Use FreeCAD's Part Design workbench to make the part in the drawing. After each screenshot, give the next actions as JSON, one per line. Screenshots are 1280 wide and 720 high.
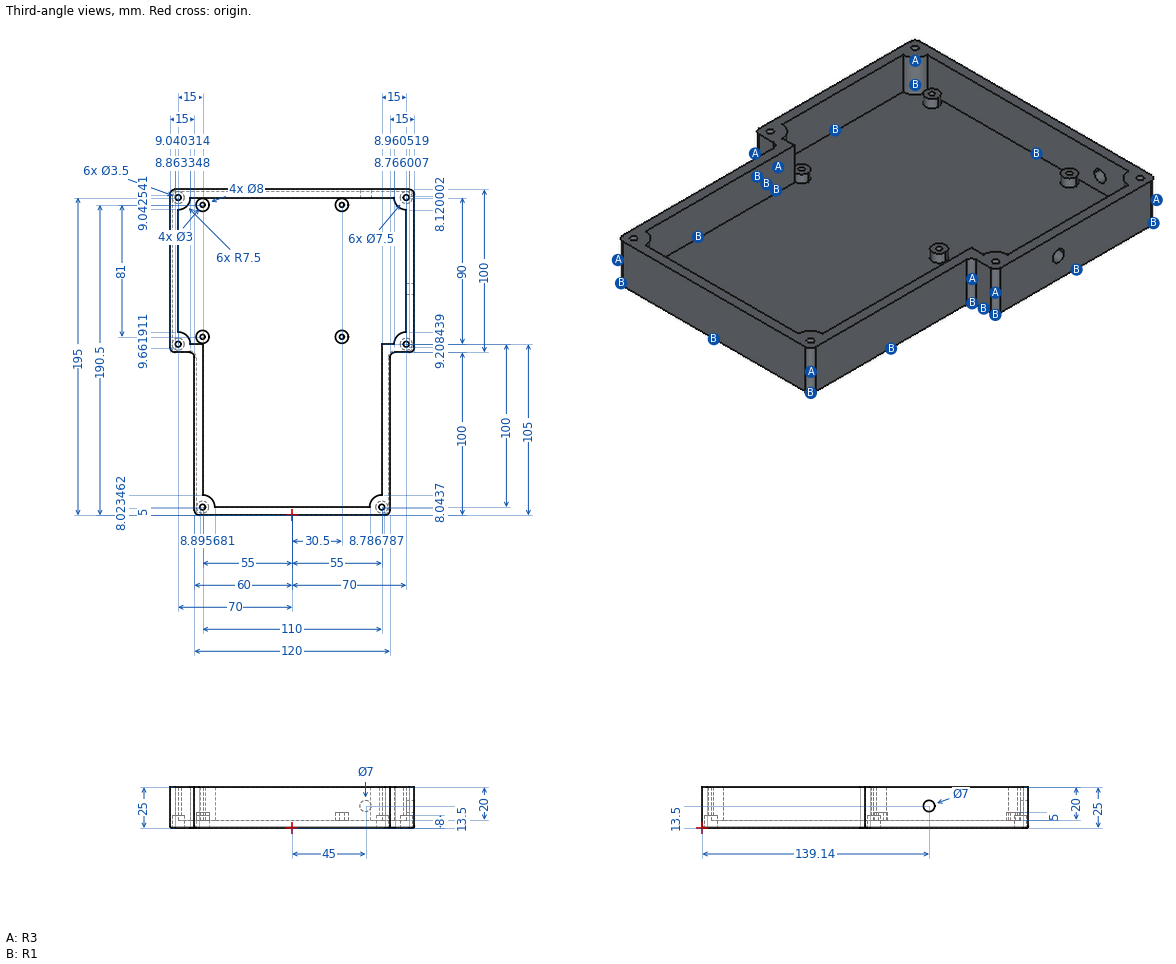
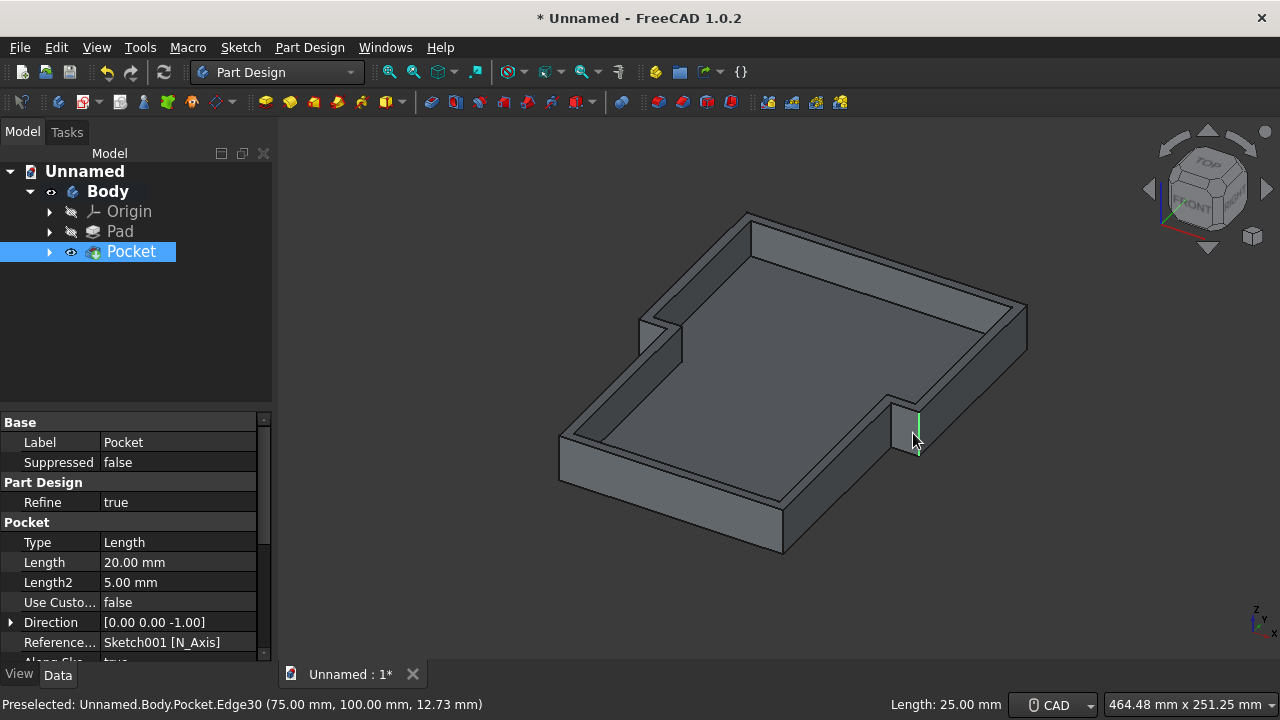
{"action": "left_click", "coordinate": [783, 531], "text": "ctrl"}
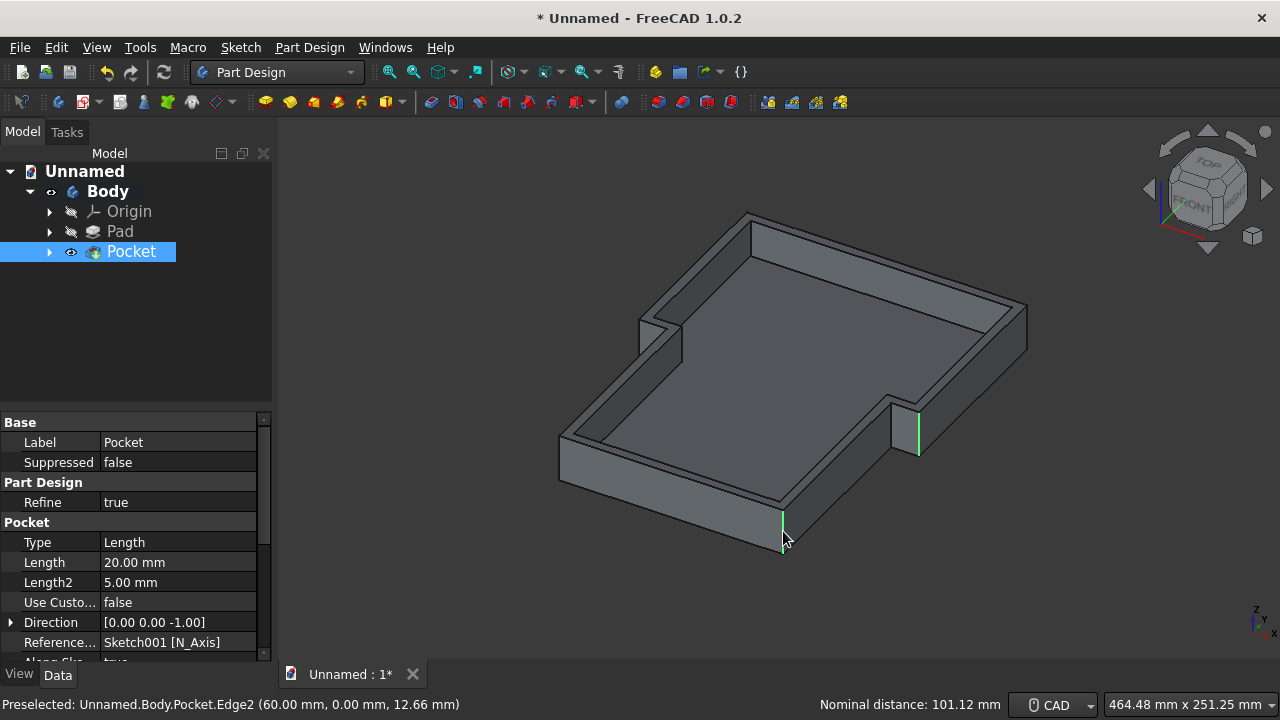
{"action": "key", "text": "0"}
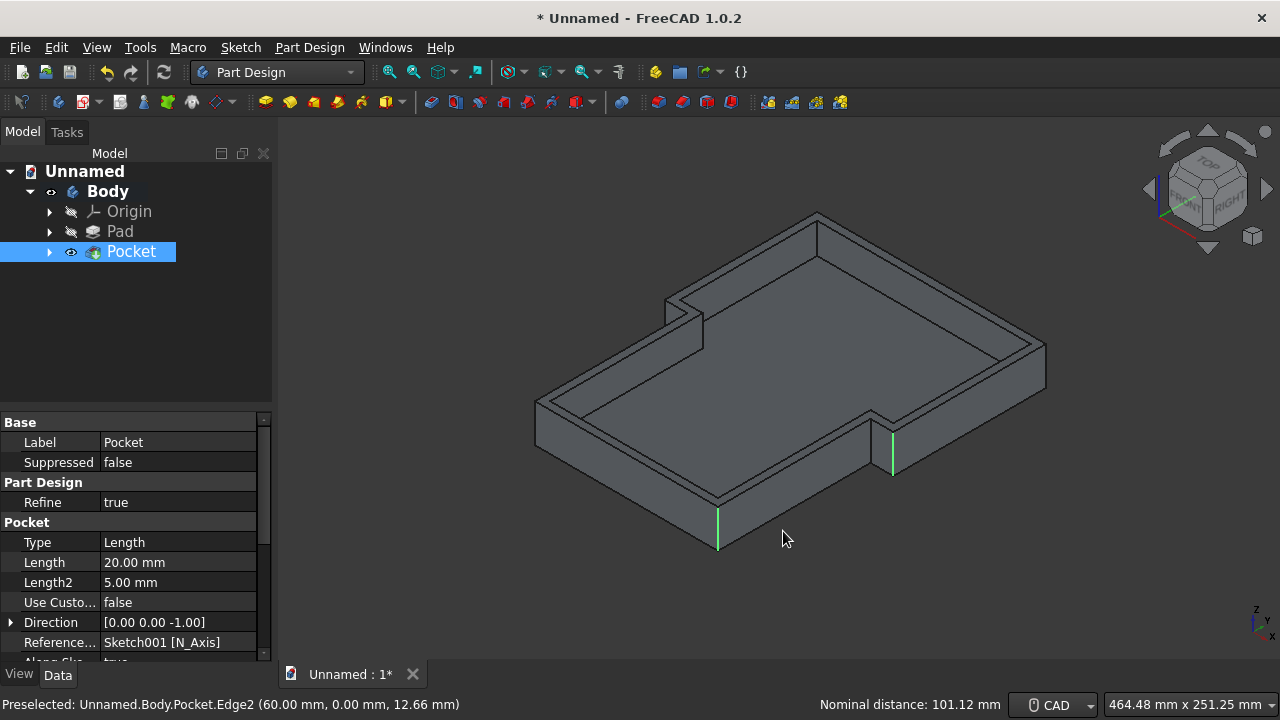
{"action": "key", "text": "2"}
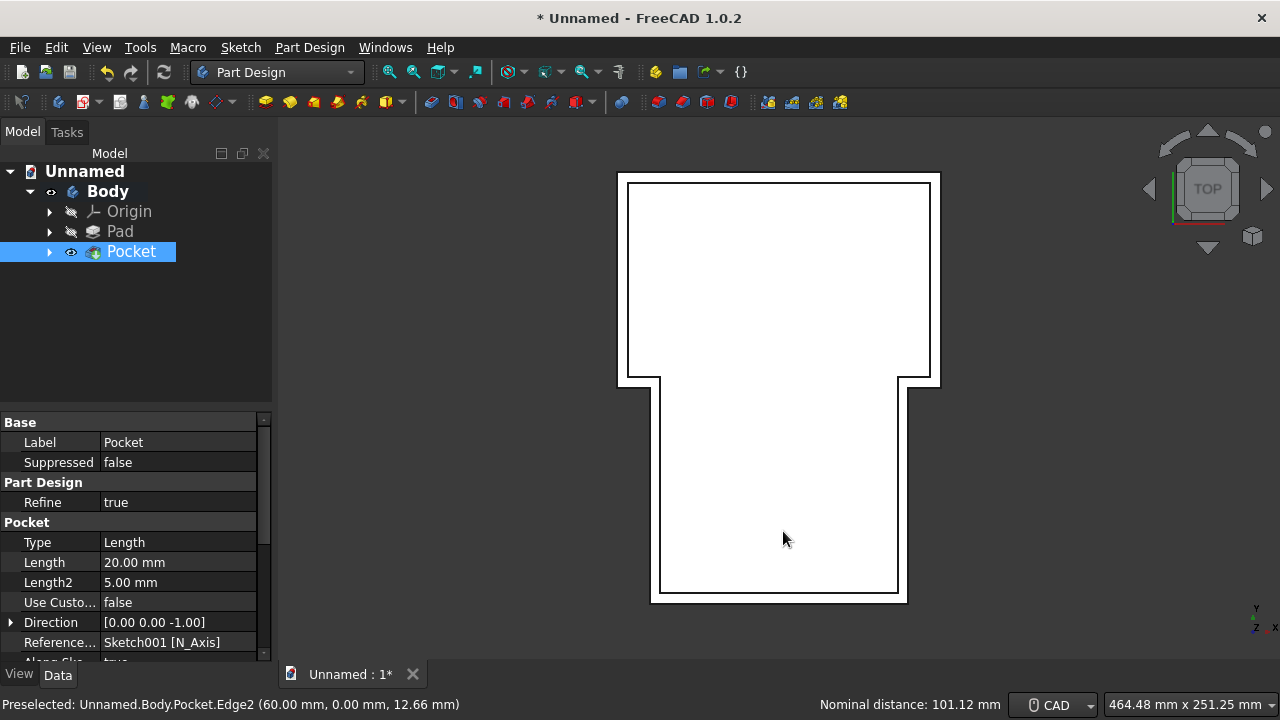
{"action": "key", "text": "1"}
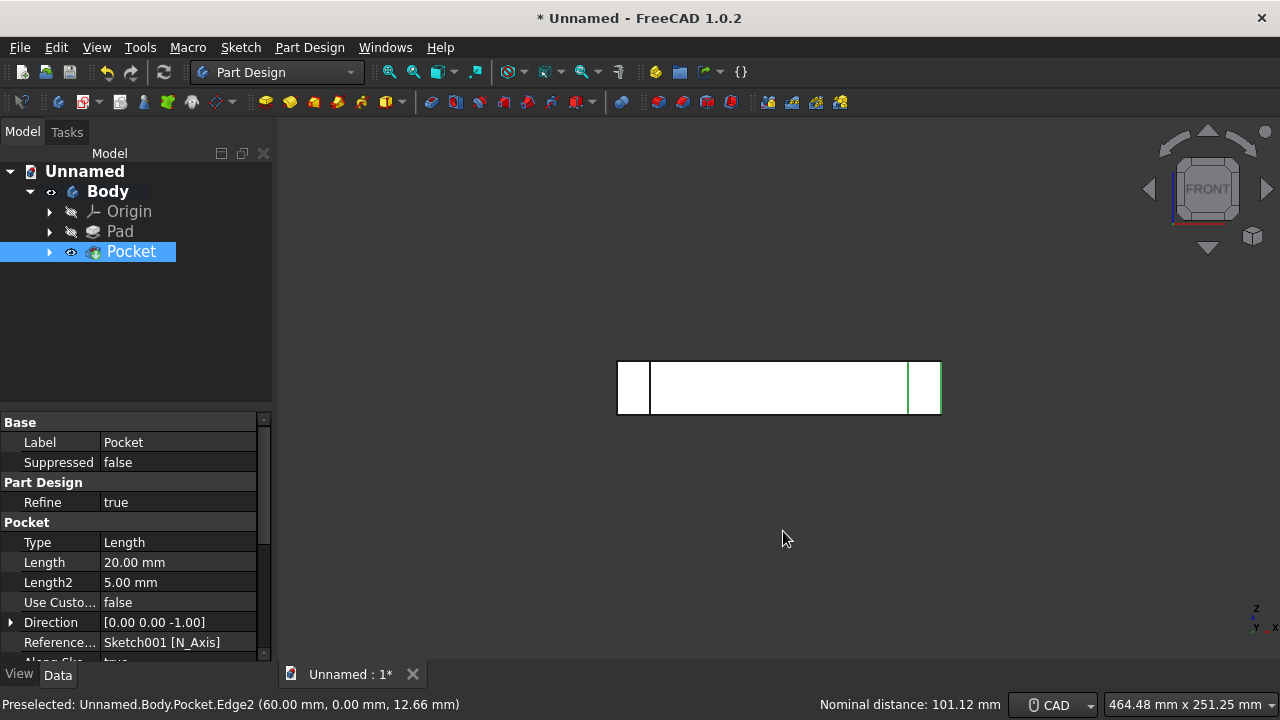
{"action": "key", "text": "v f"}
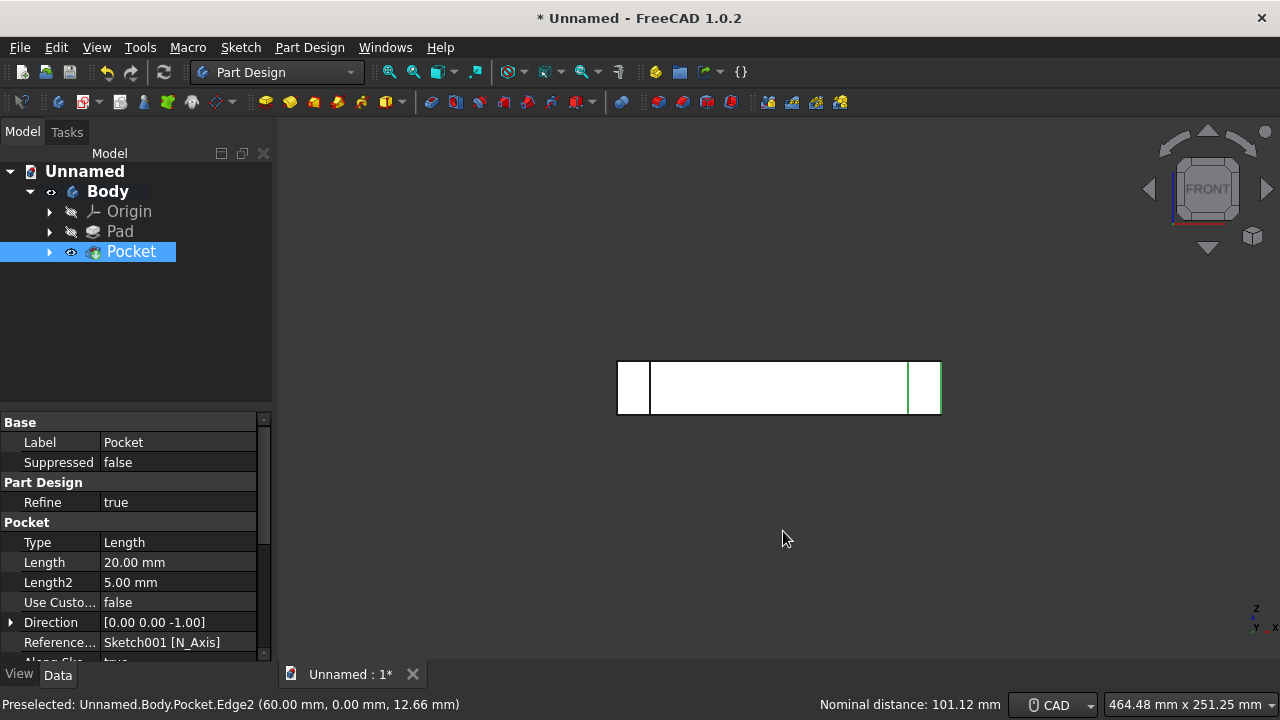
{"action": "left_click", "coordinate": [617, 387], "text": "ctrl"}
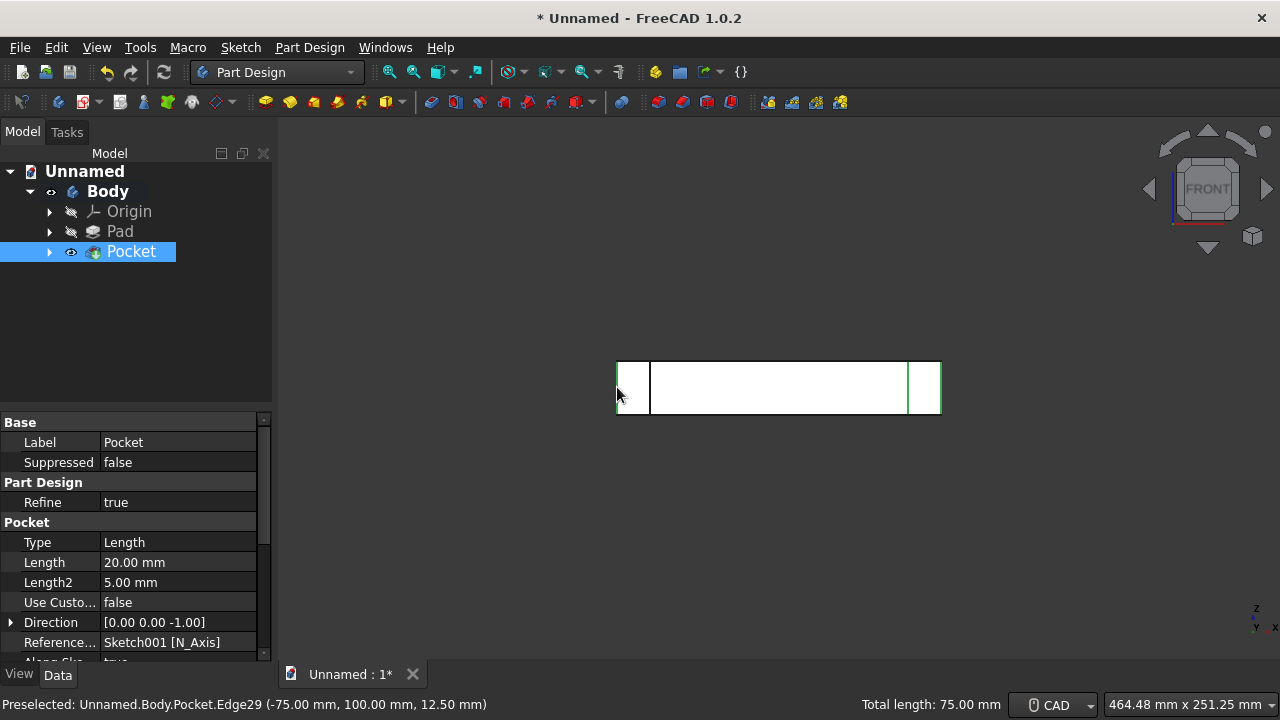
{"action": "left_click", "coordinate": [650, 387], "text": "ctrl"}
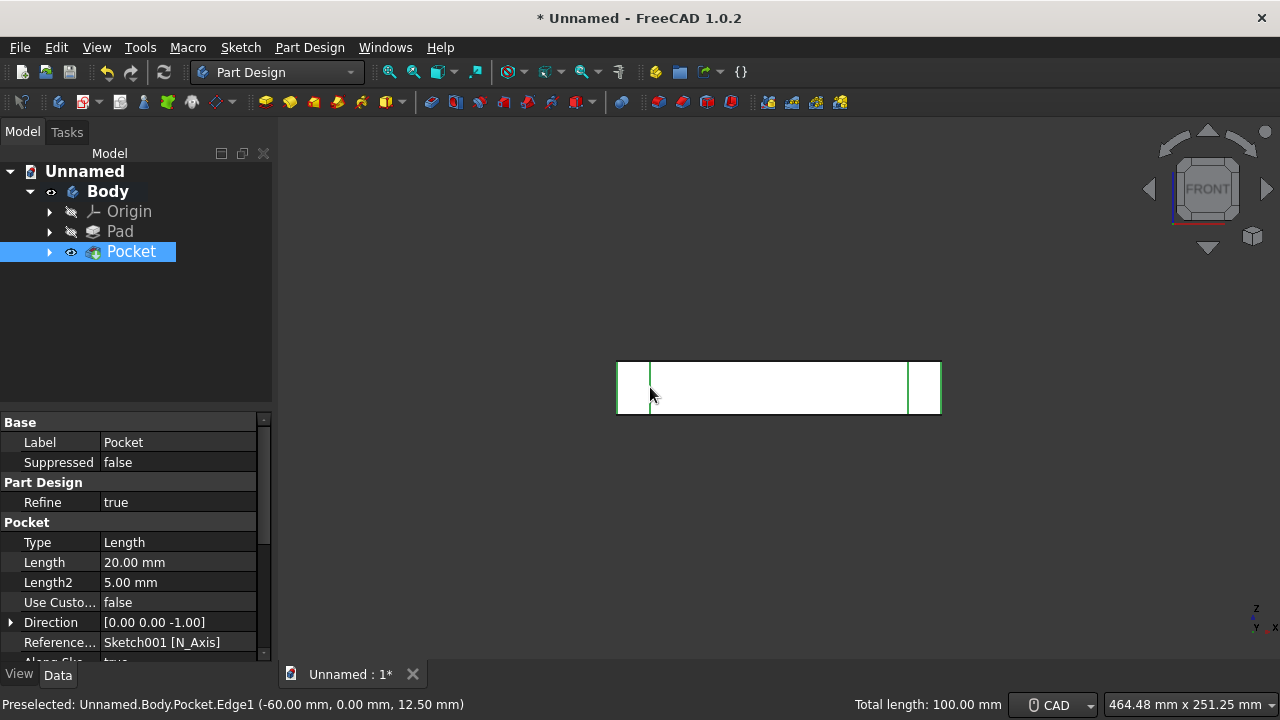
{"action": "key", "text": "3"}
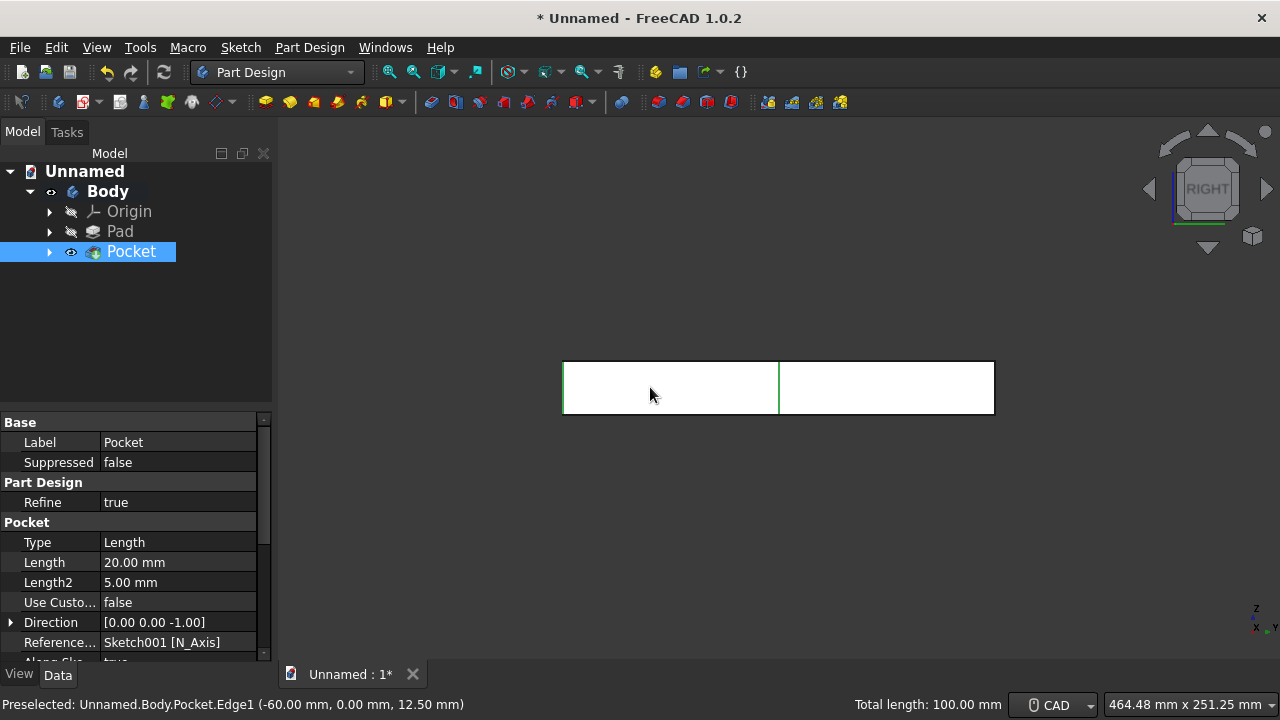
{"action": "left_click", "coordinate": [390, 72]}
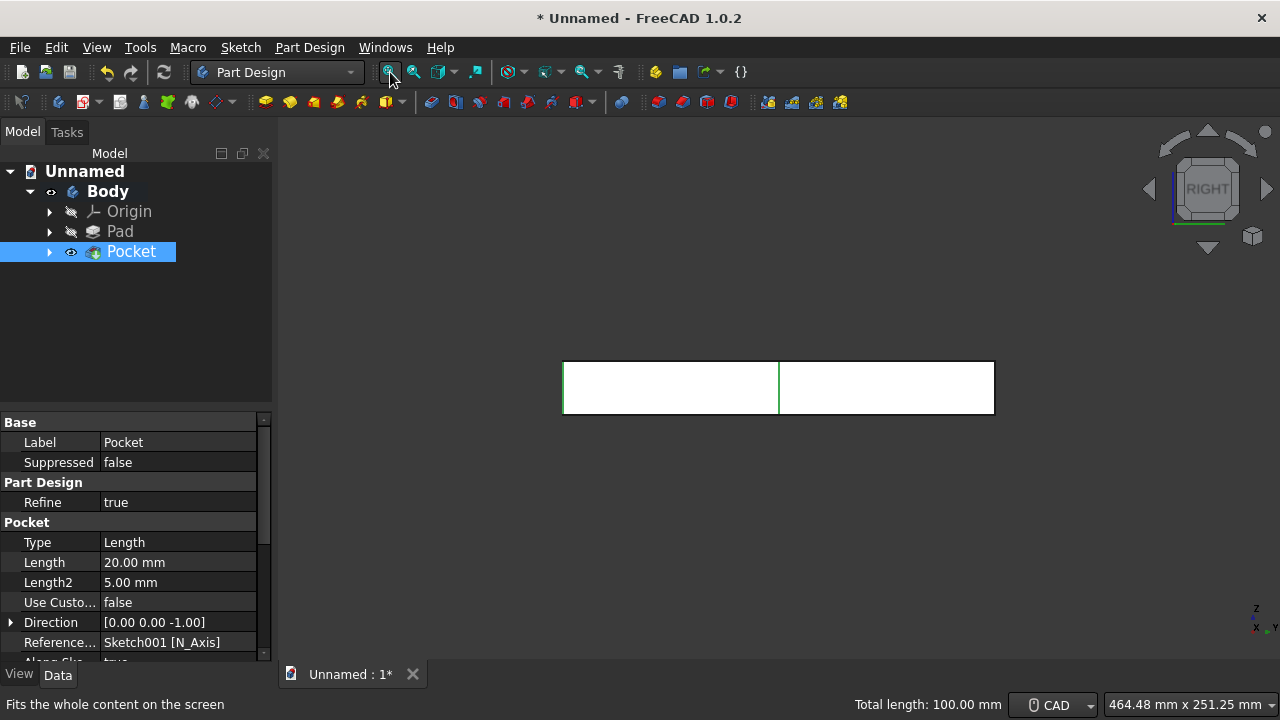
{"action": "left_click", "coordinate": [995, 387], "text": "ctrl"}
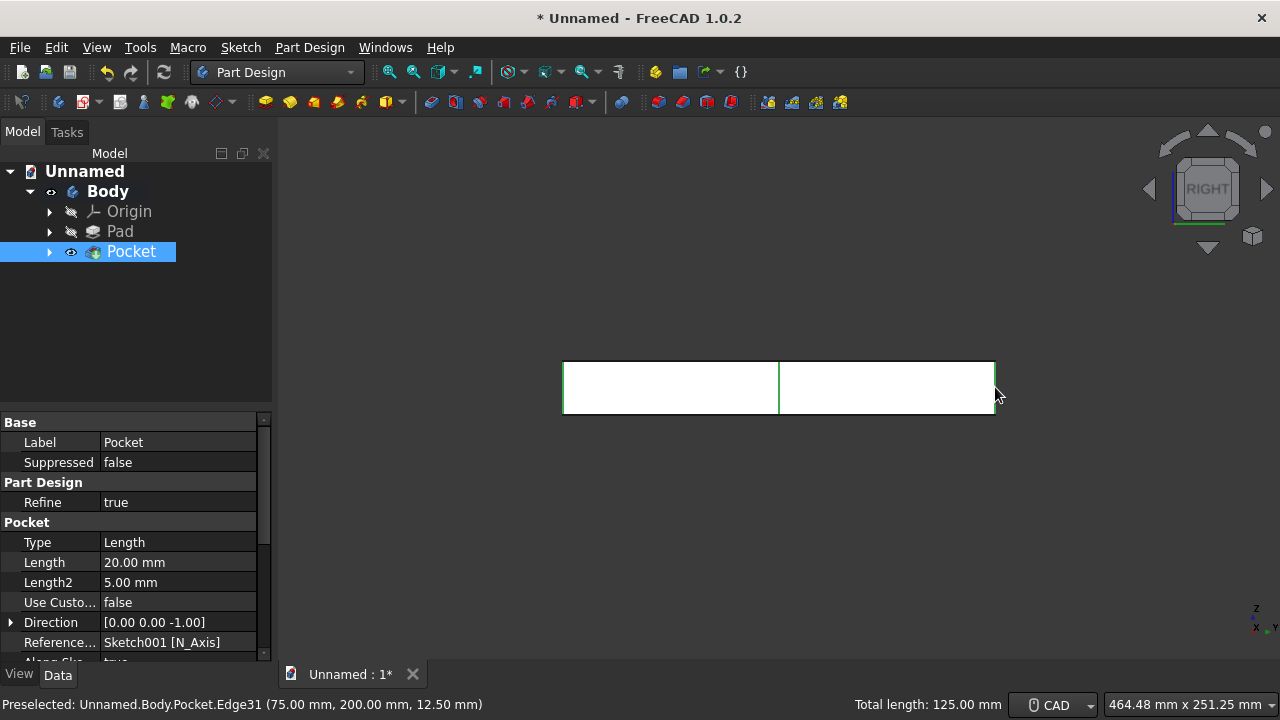
{"action": "key", "text": "5"}